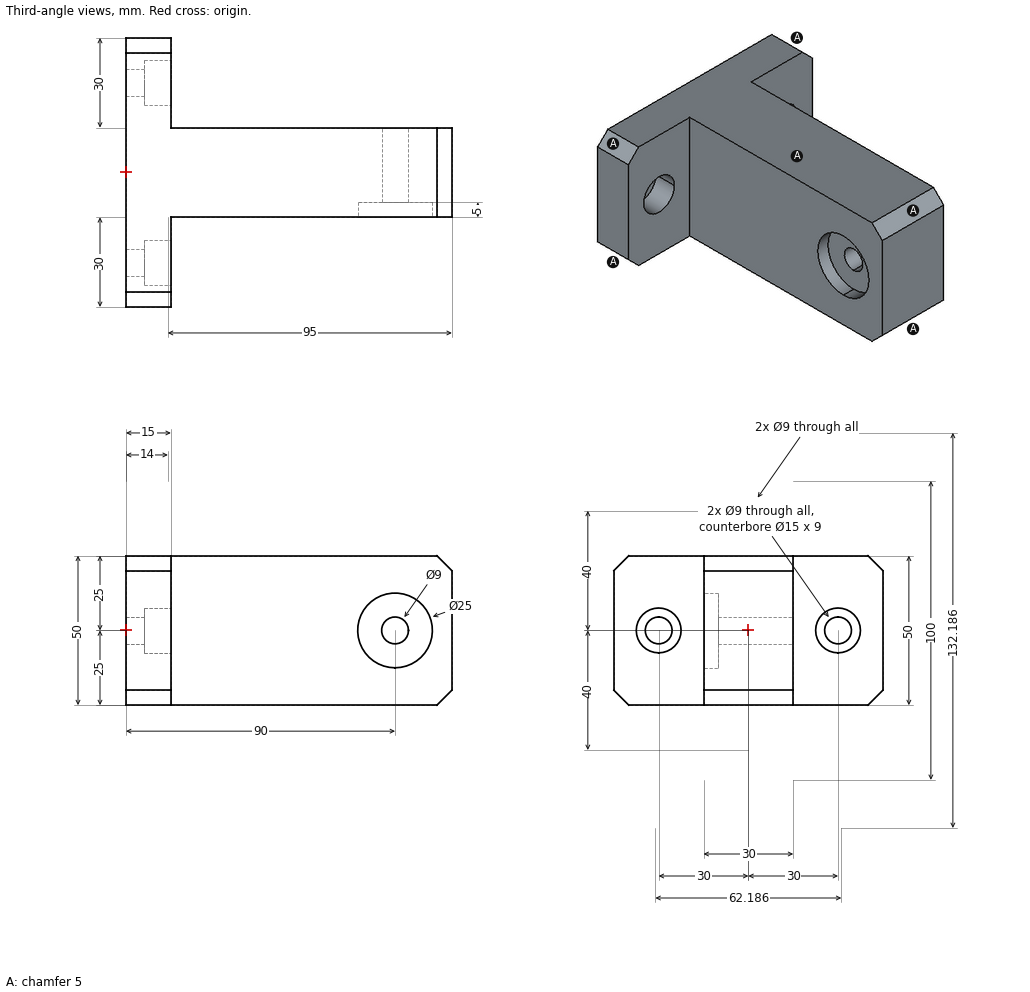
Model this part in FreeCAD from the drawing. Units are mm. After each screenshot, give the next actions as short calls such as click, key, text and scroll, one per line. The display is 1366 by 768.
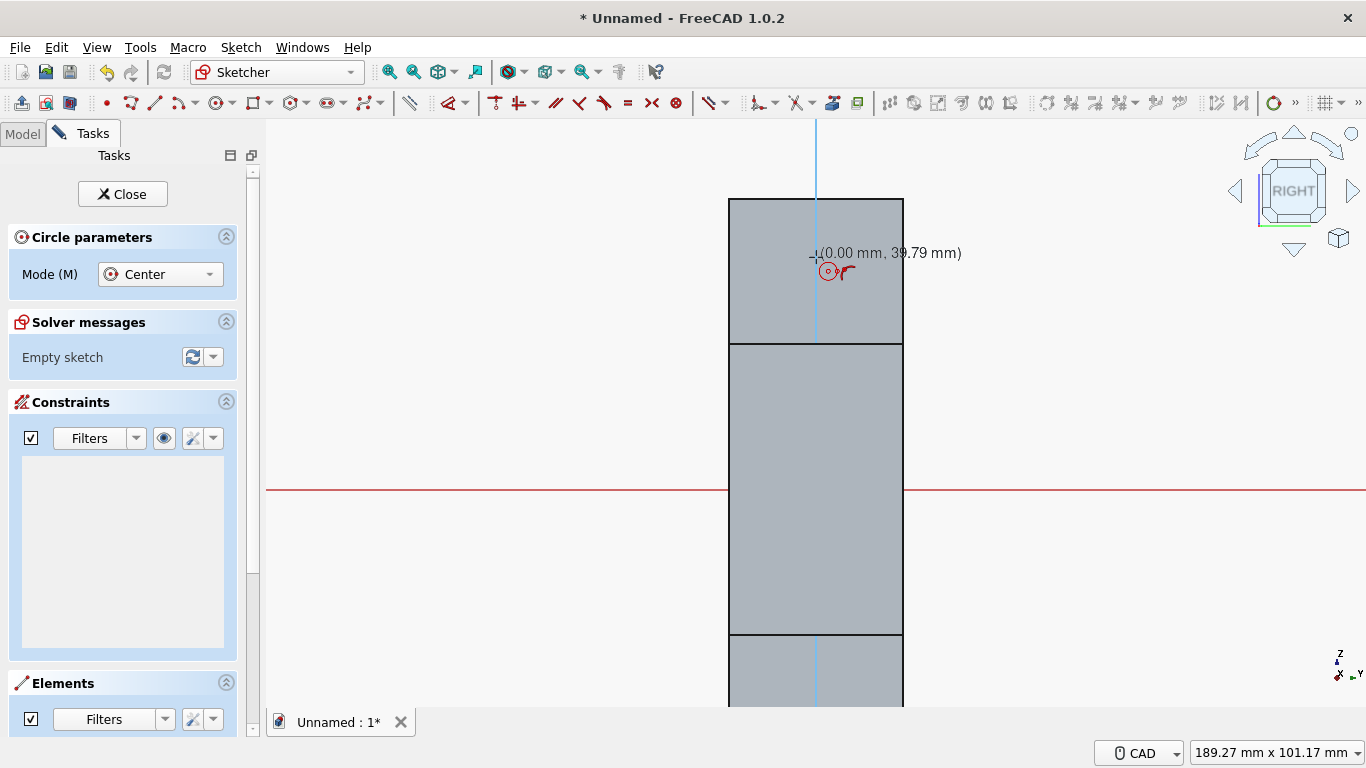
click(816, 257)
move(834, 239)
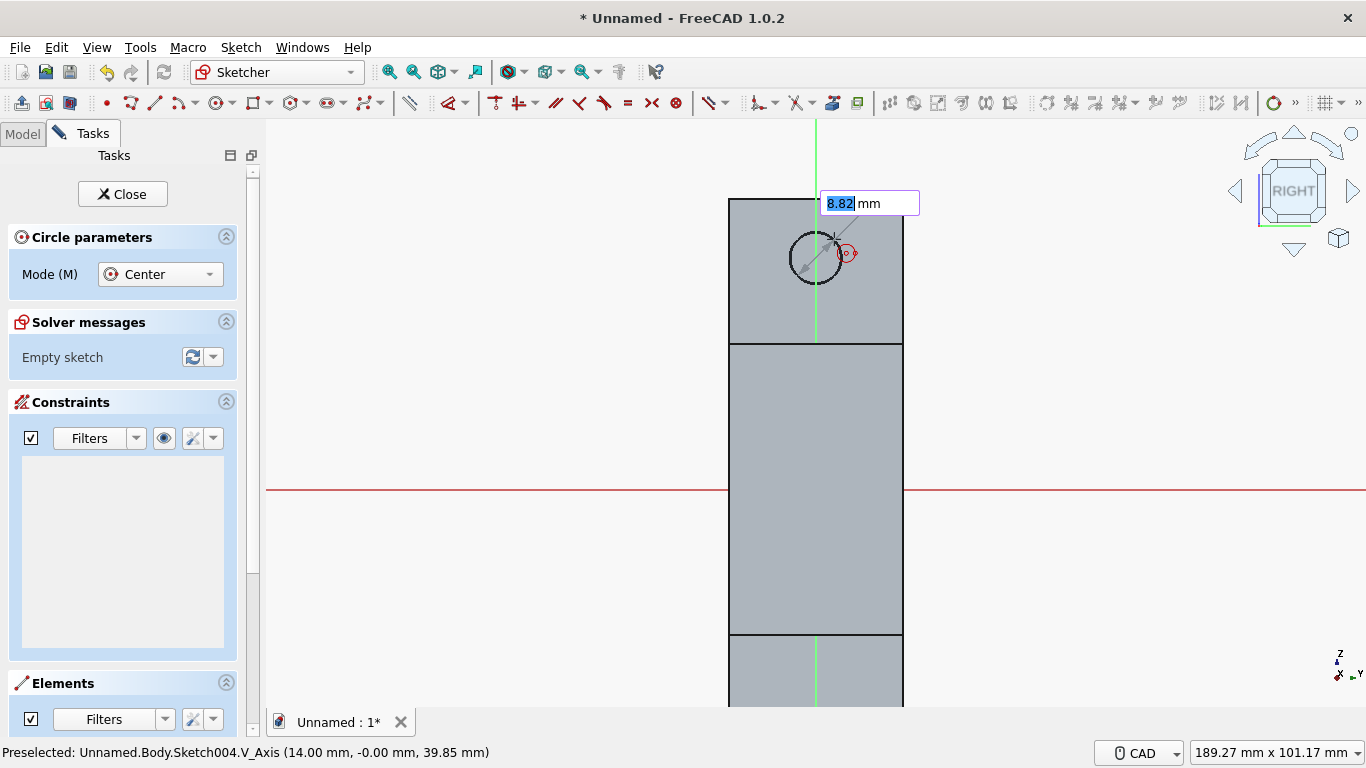
text(9)
key(Return)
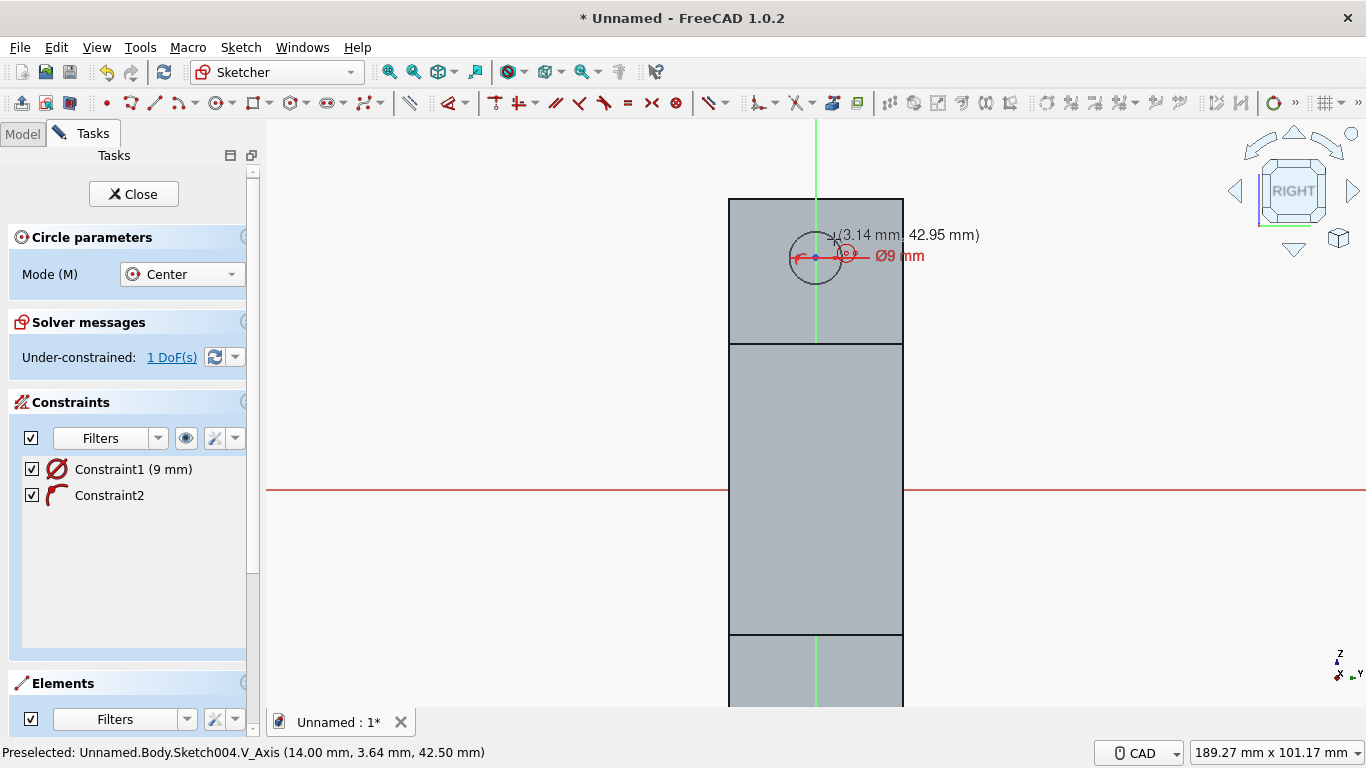
scroll(609, 257, down, 2)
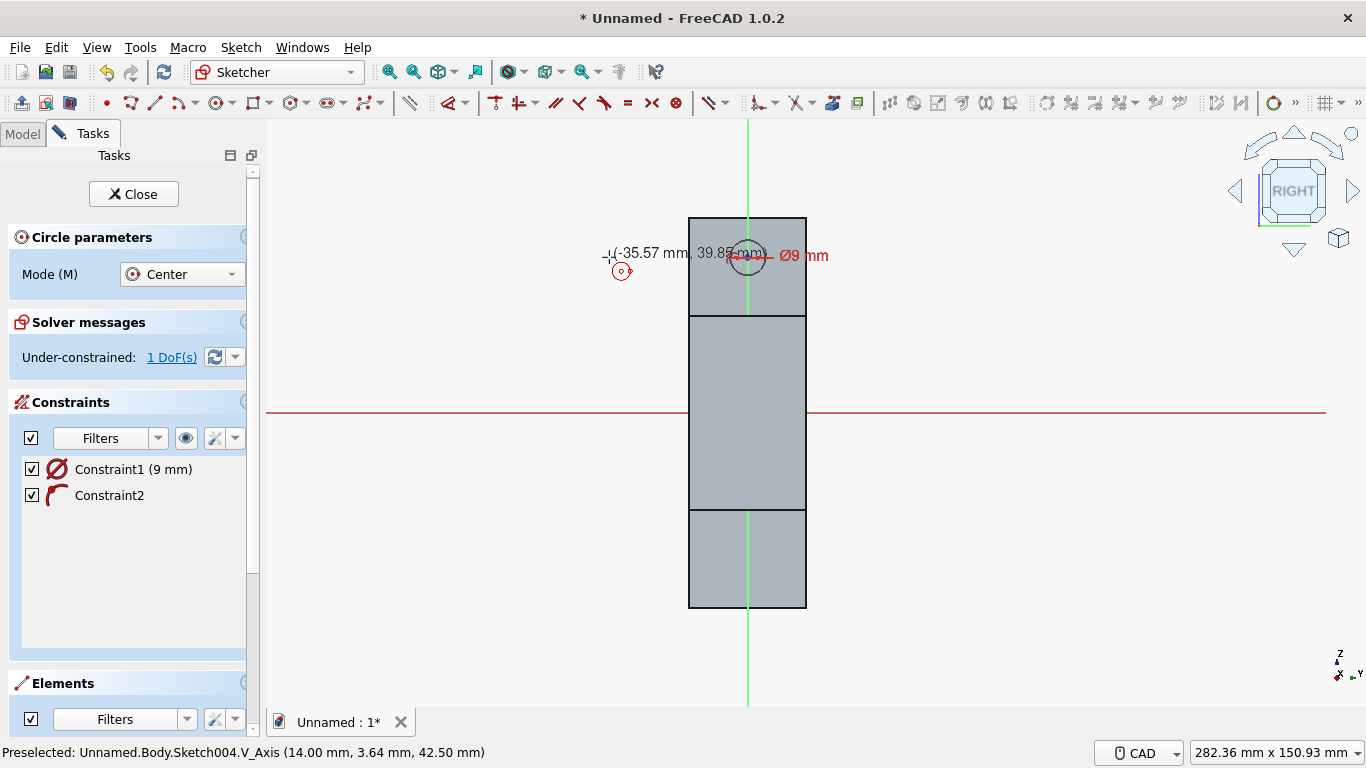
scroll(748, 569, up, 2)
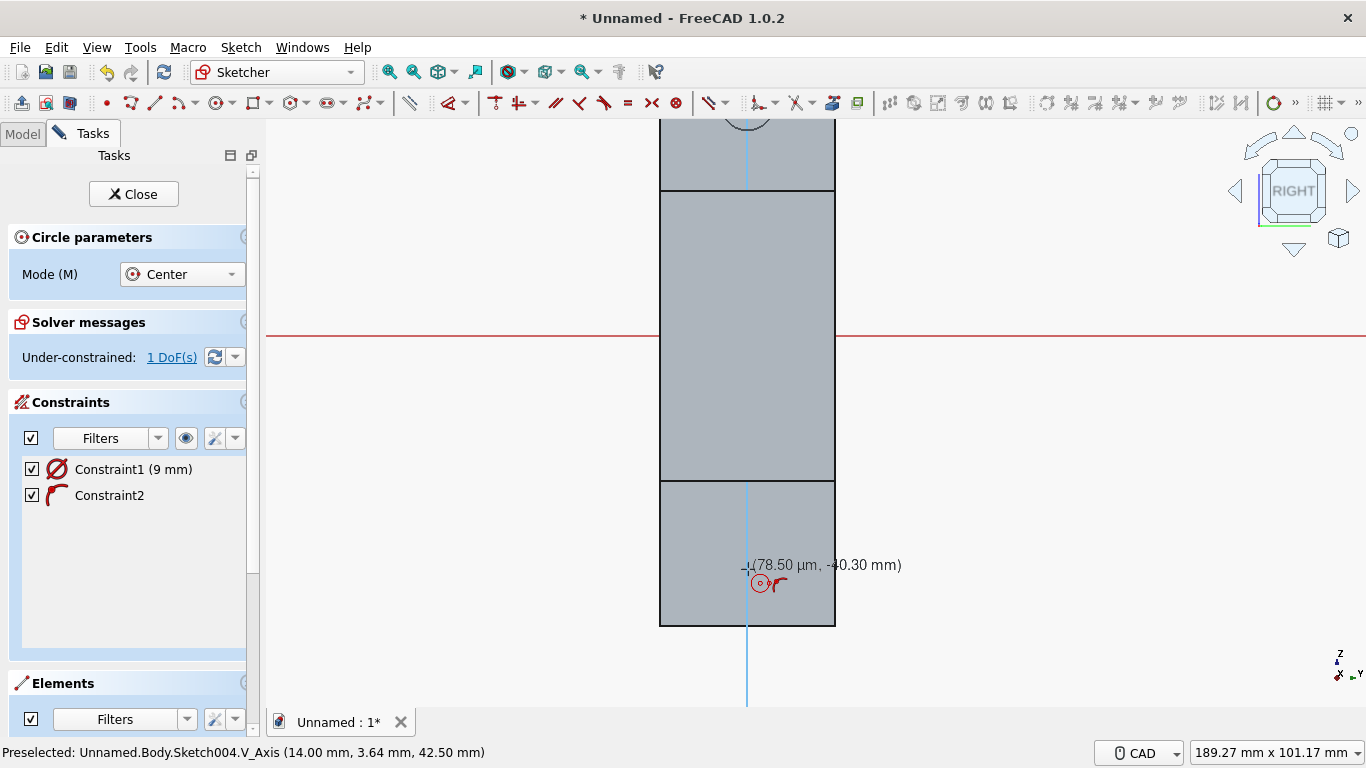
click(747, 568)
move(766, 550)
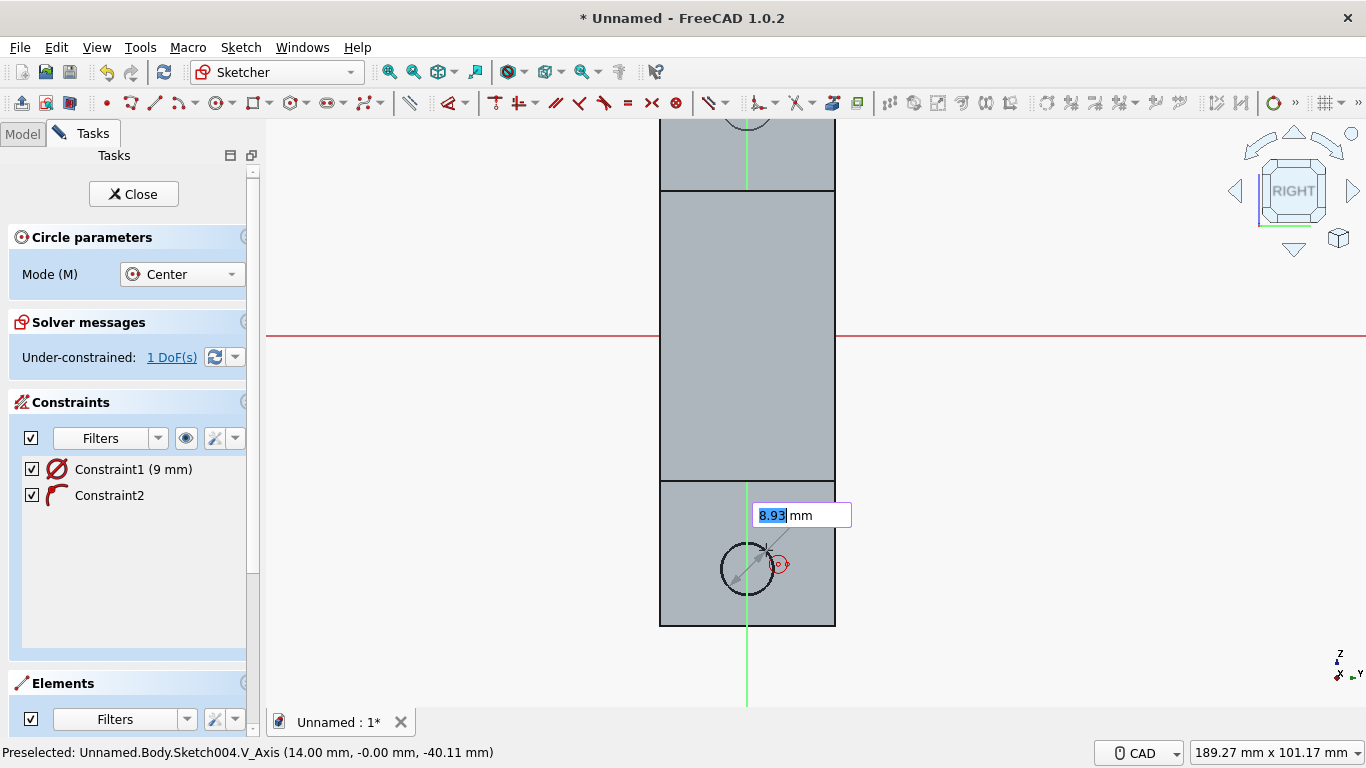
text(9)
key(Return)
key(Escape)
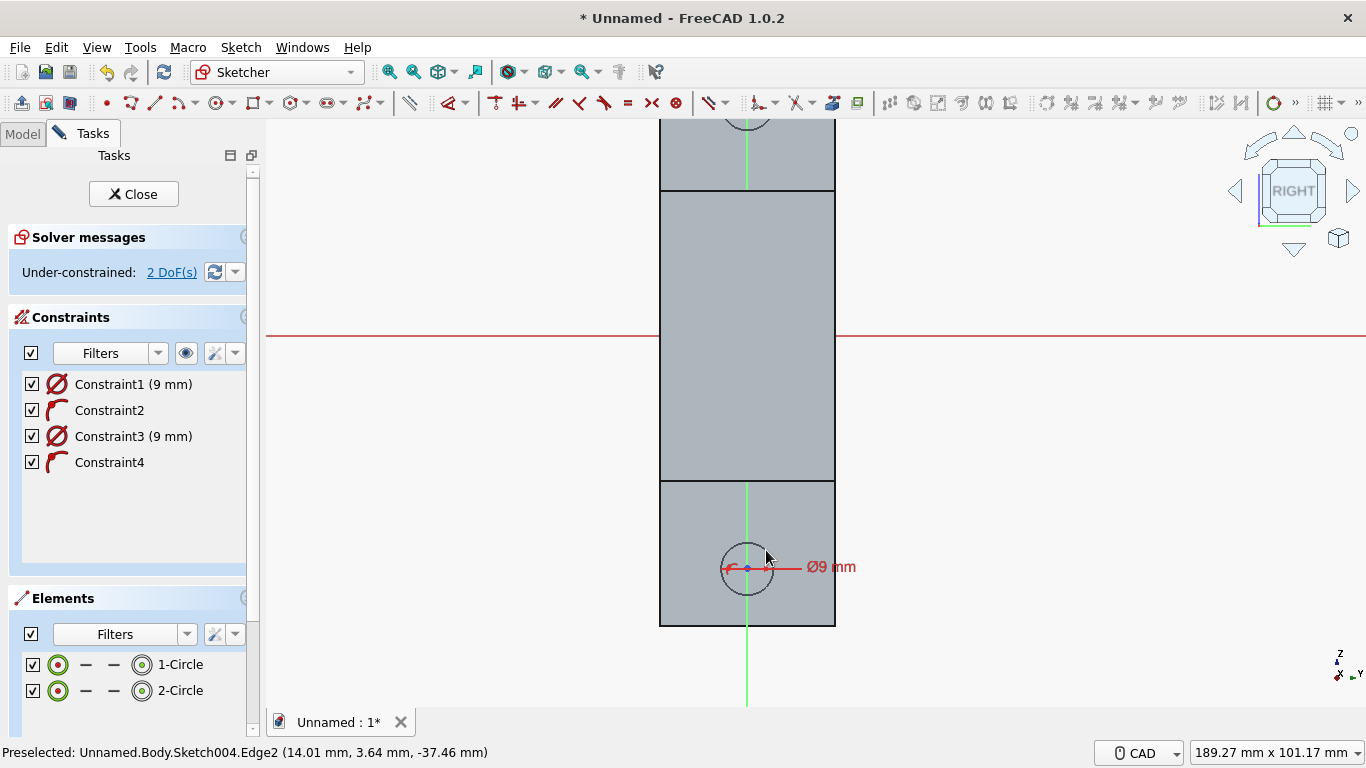
click(448, 104)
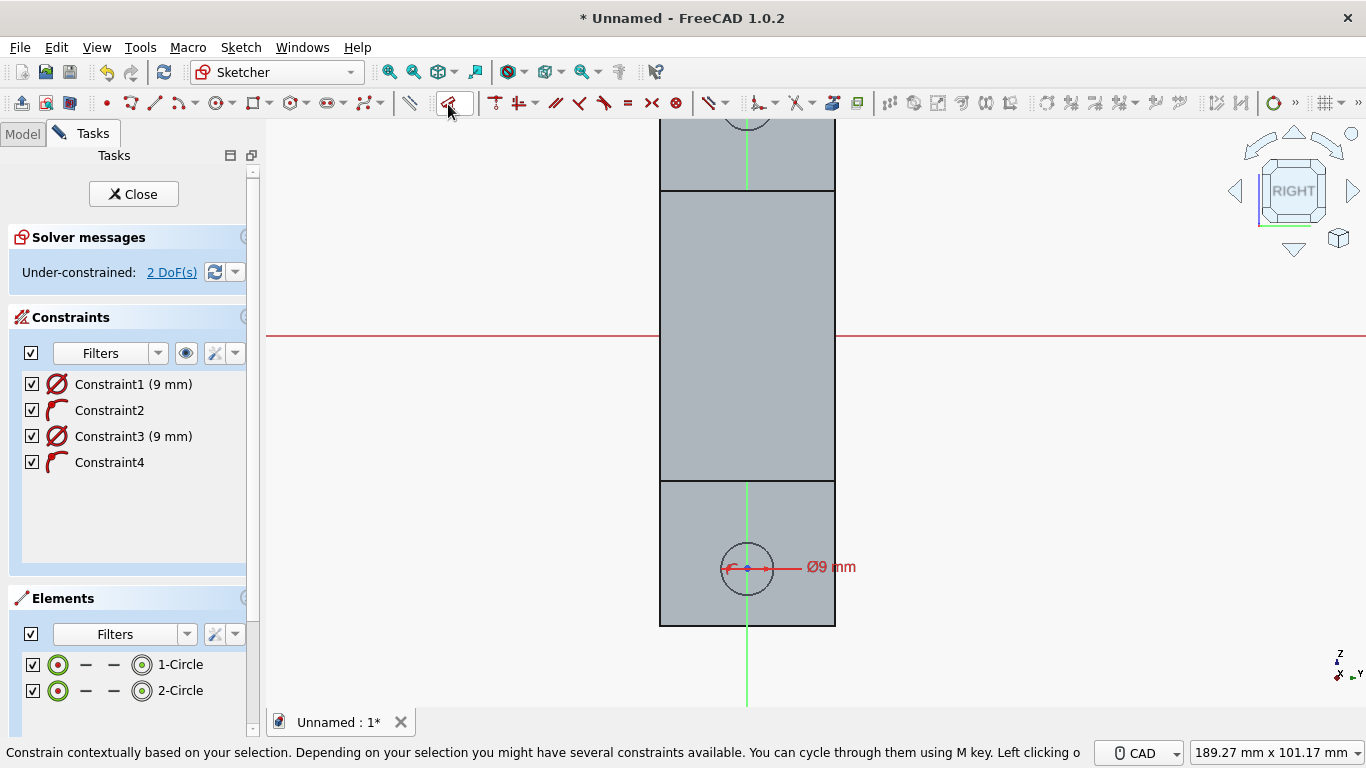
scroll(748, 570, down, 2)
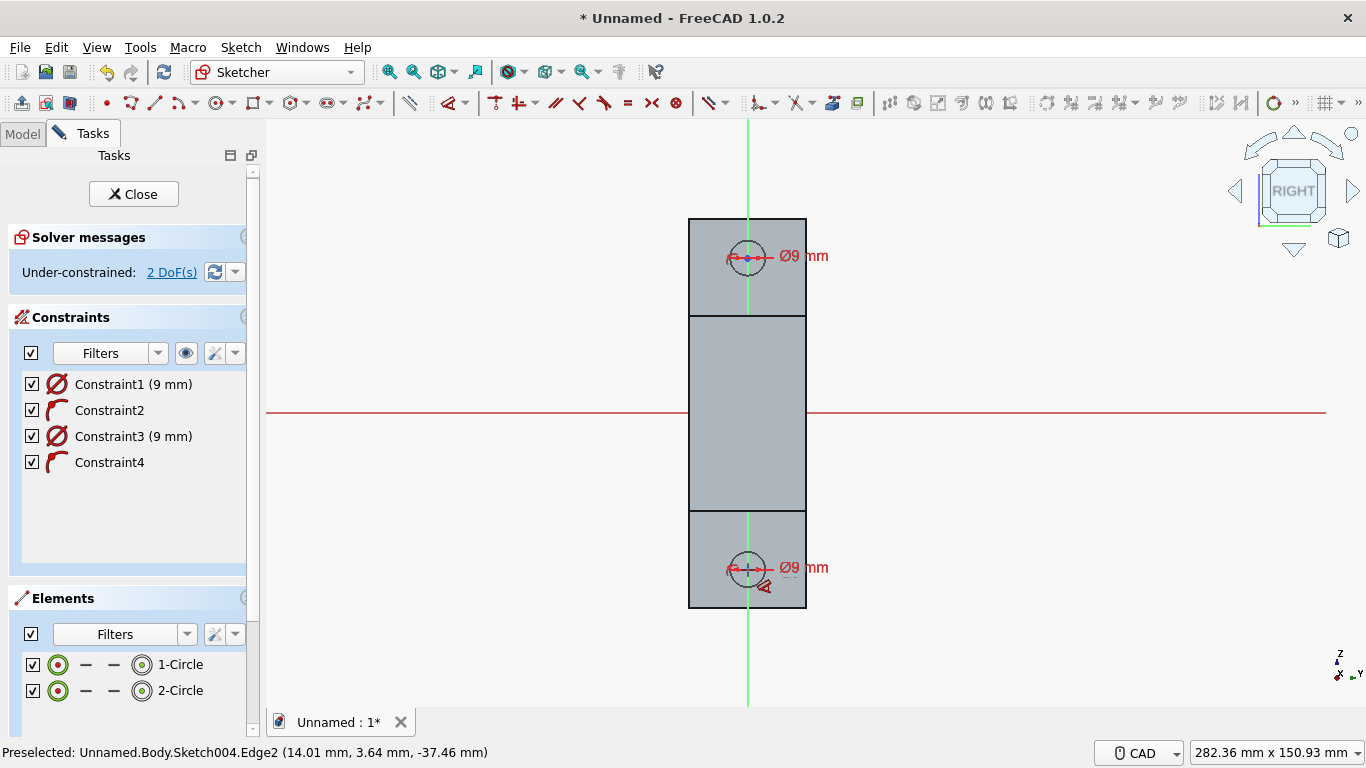
click(748, 258)
click(782, 336)